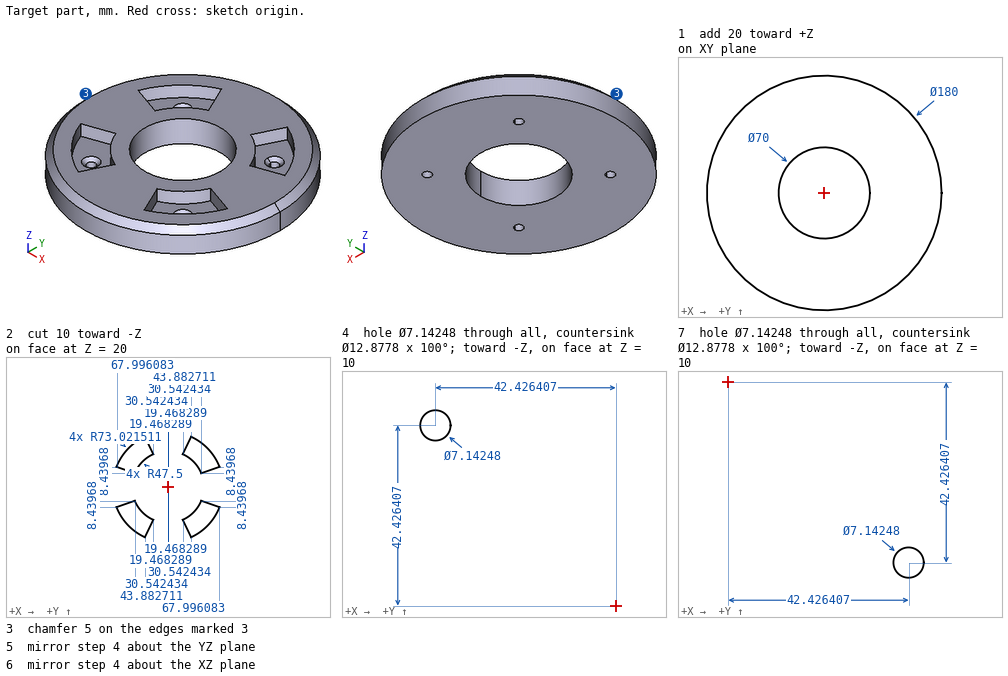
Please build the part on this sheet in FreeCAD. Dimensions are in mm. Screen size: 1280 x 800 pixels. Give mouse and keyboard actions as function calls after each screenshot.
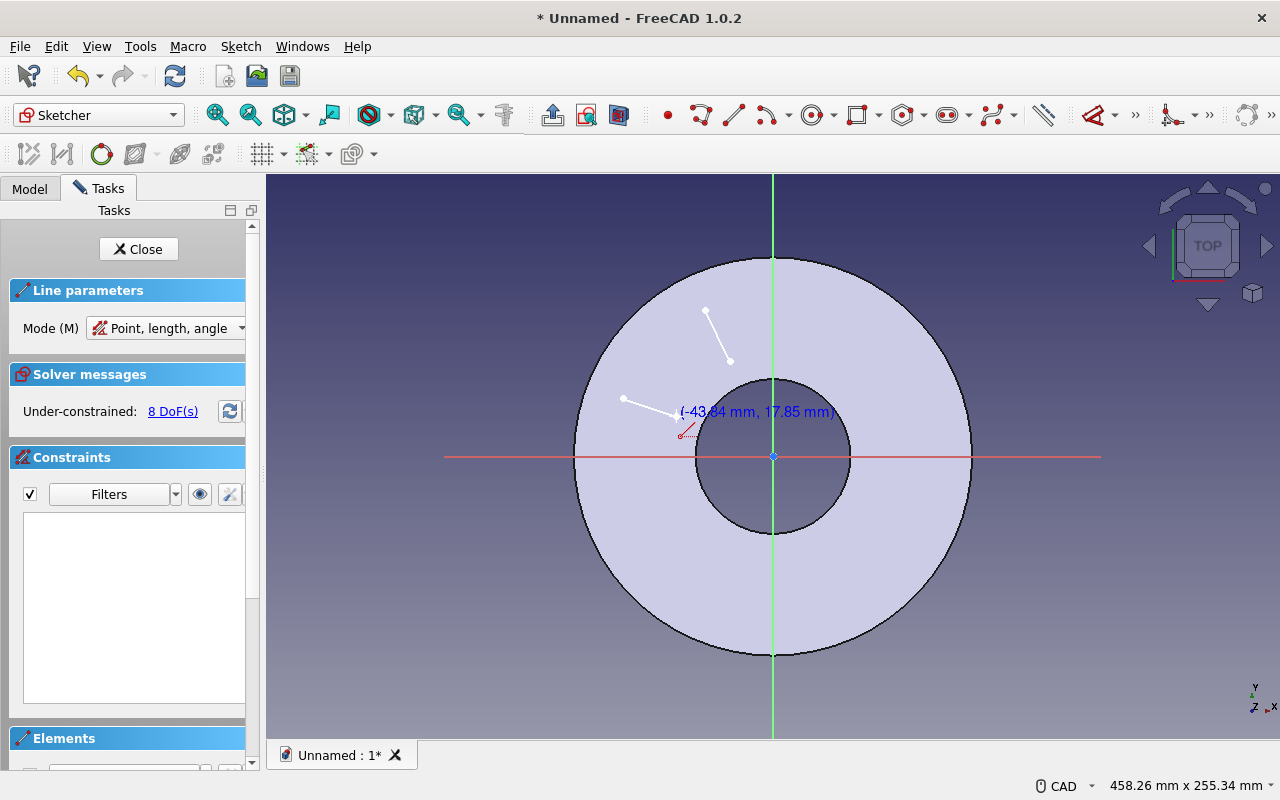
key(g)
key(3)
key(a)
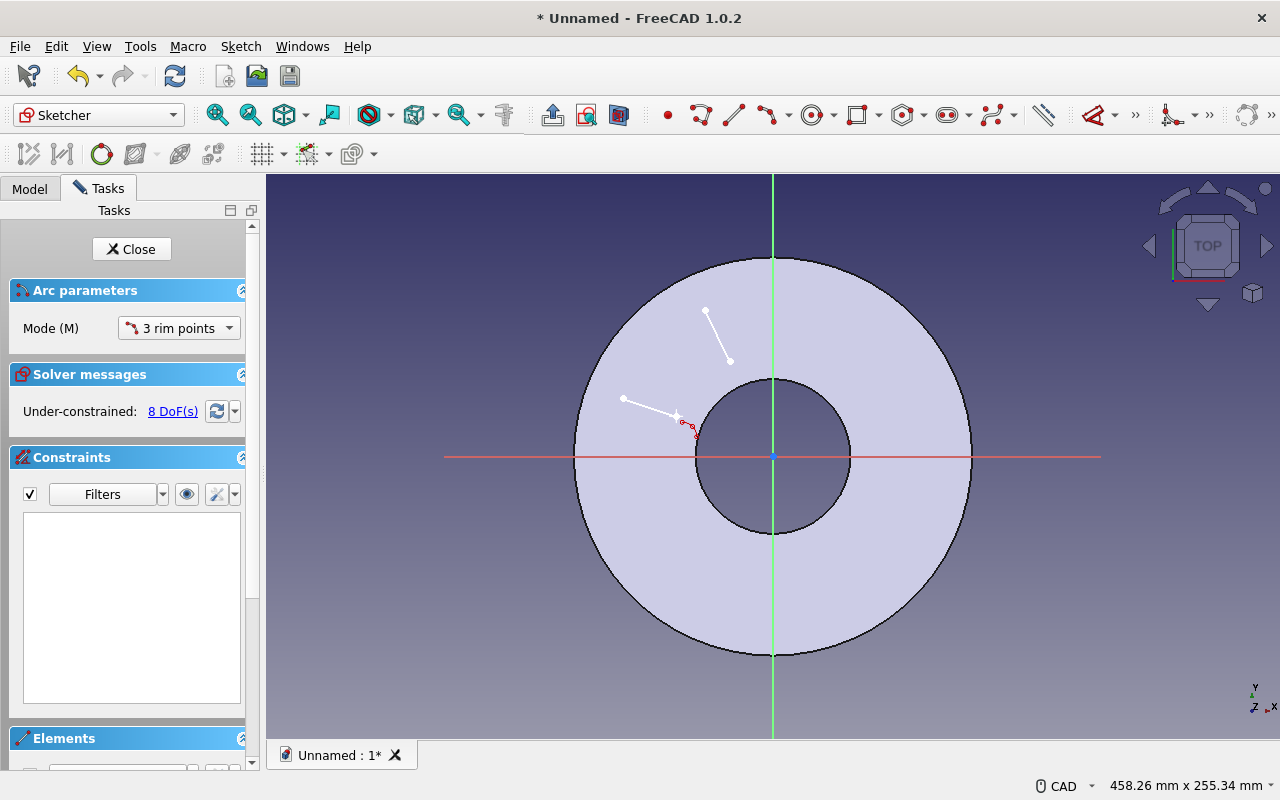
click(705, 311)
click(623, 399)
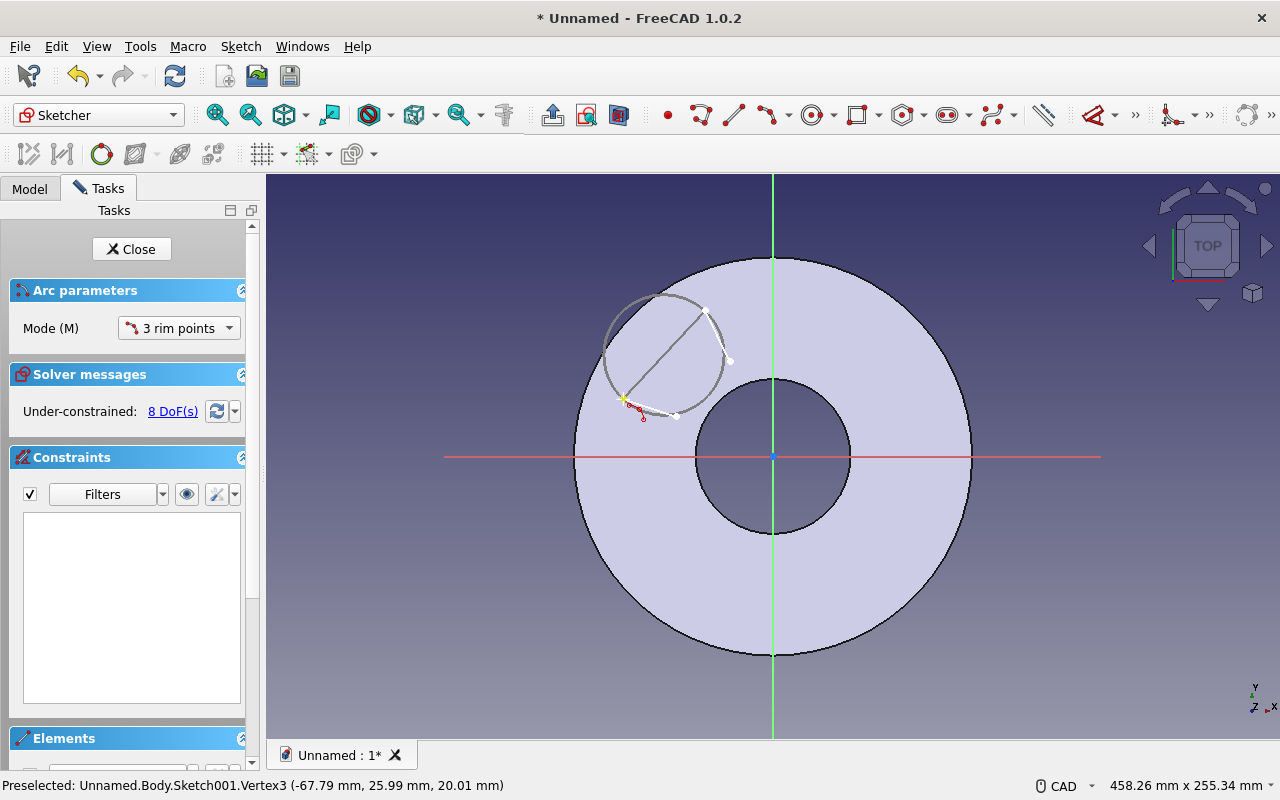
scroll(655, 346, up, 2)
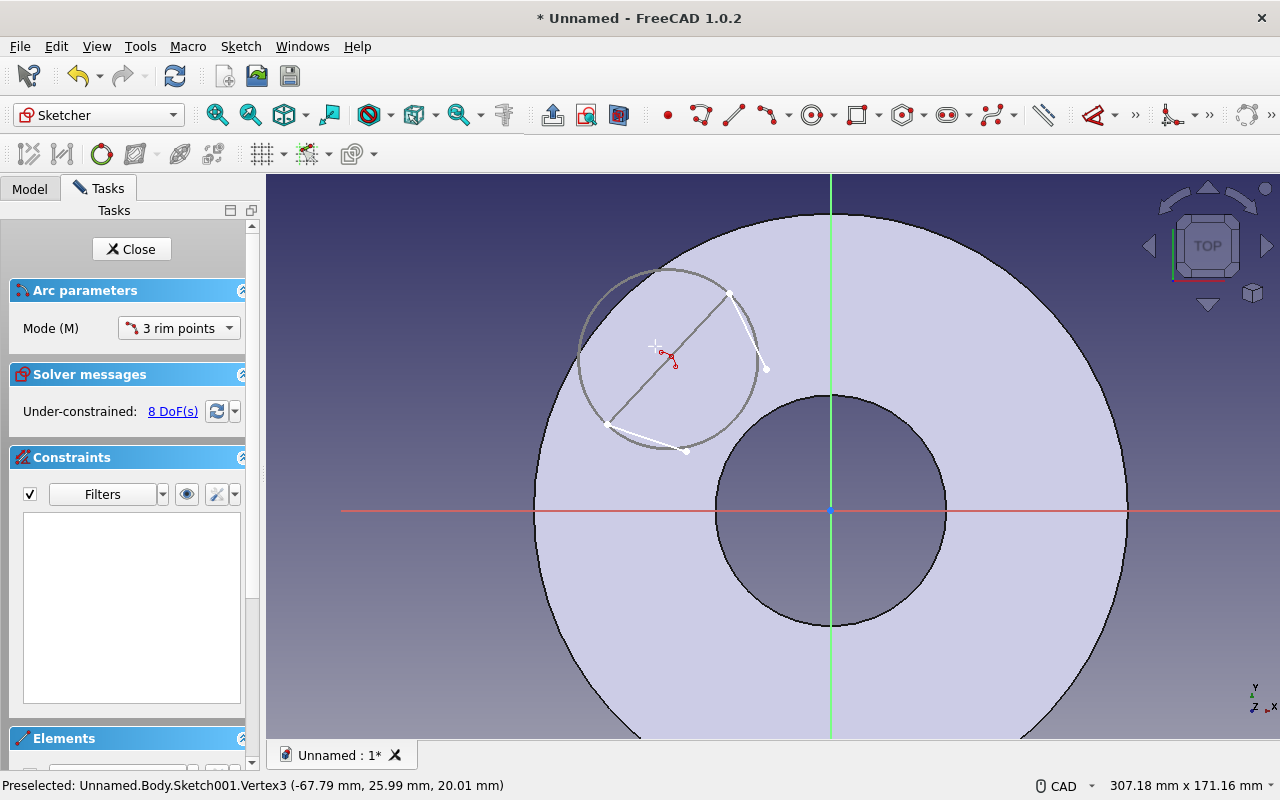
click(656, 345)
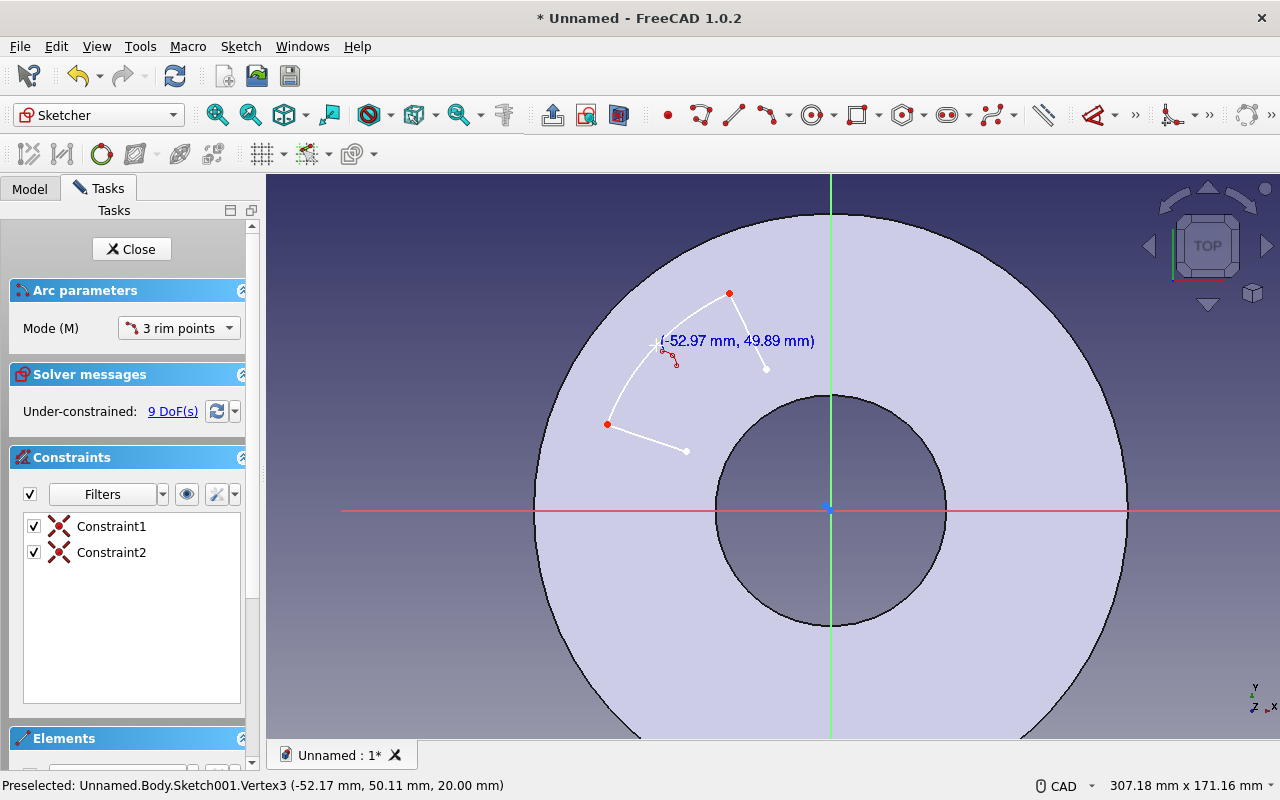
click(686, 452)
click(767, 370)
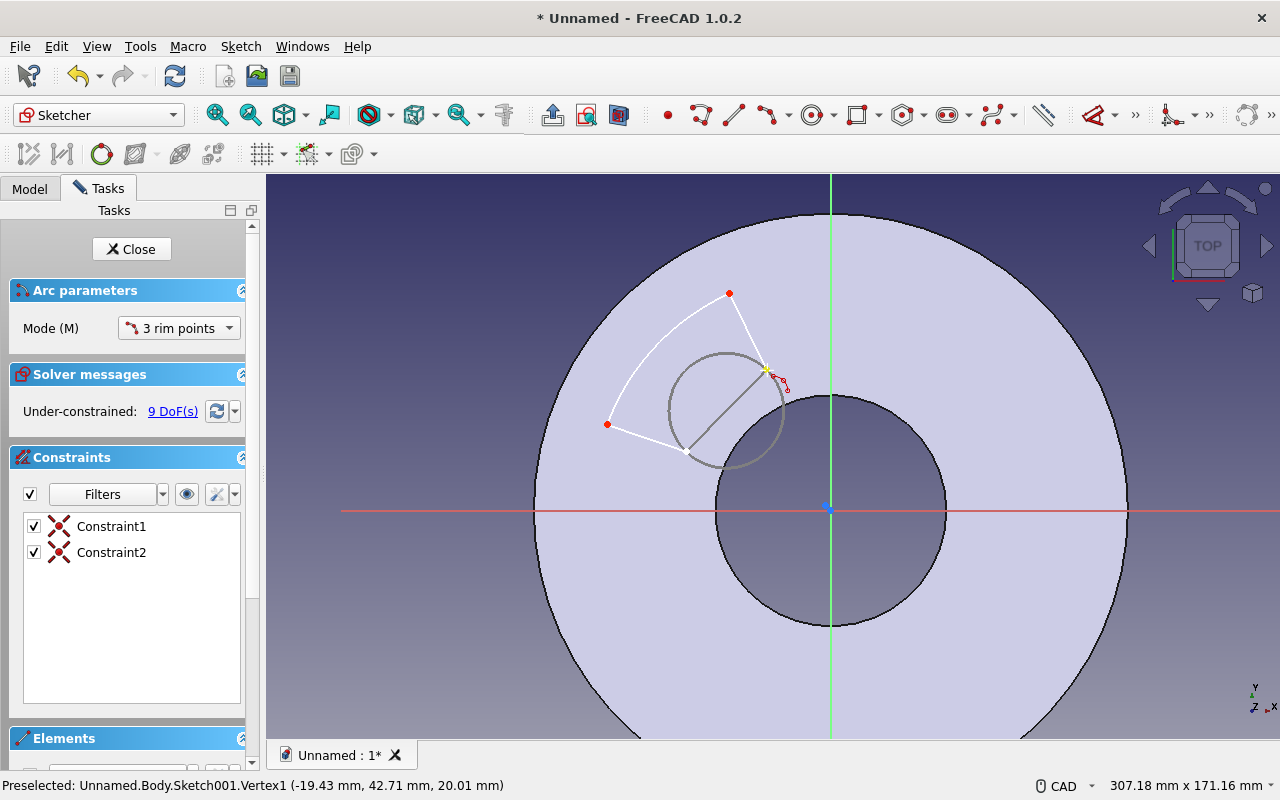
scroll(718, 401, up, 2)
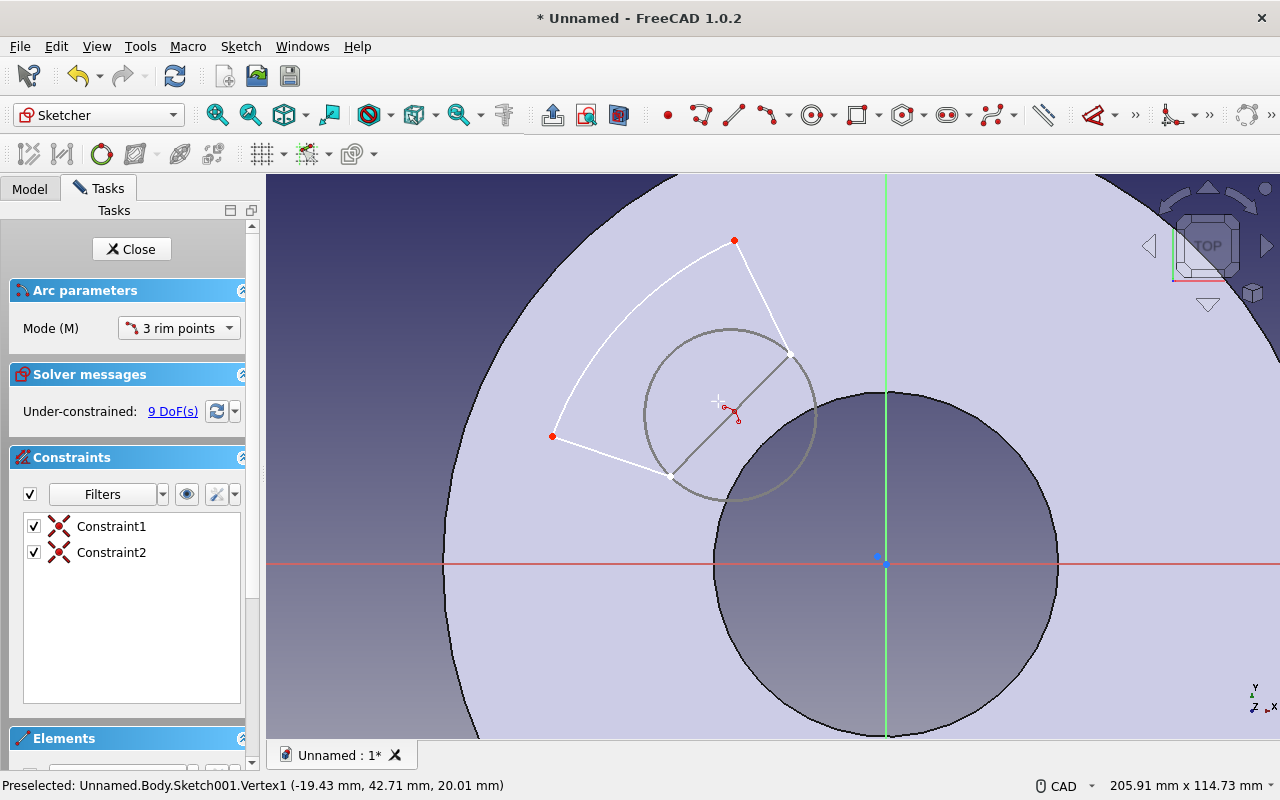
click(718, 402)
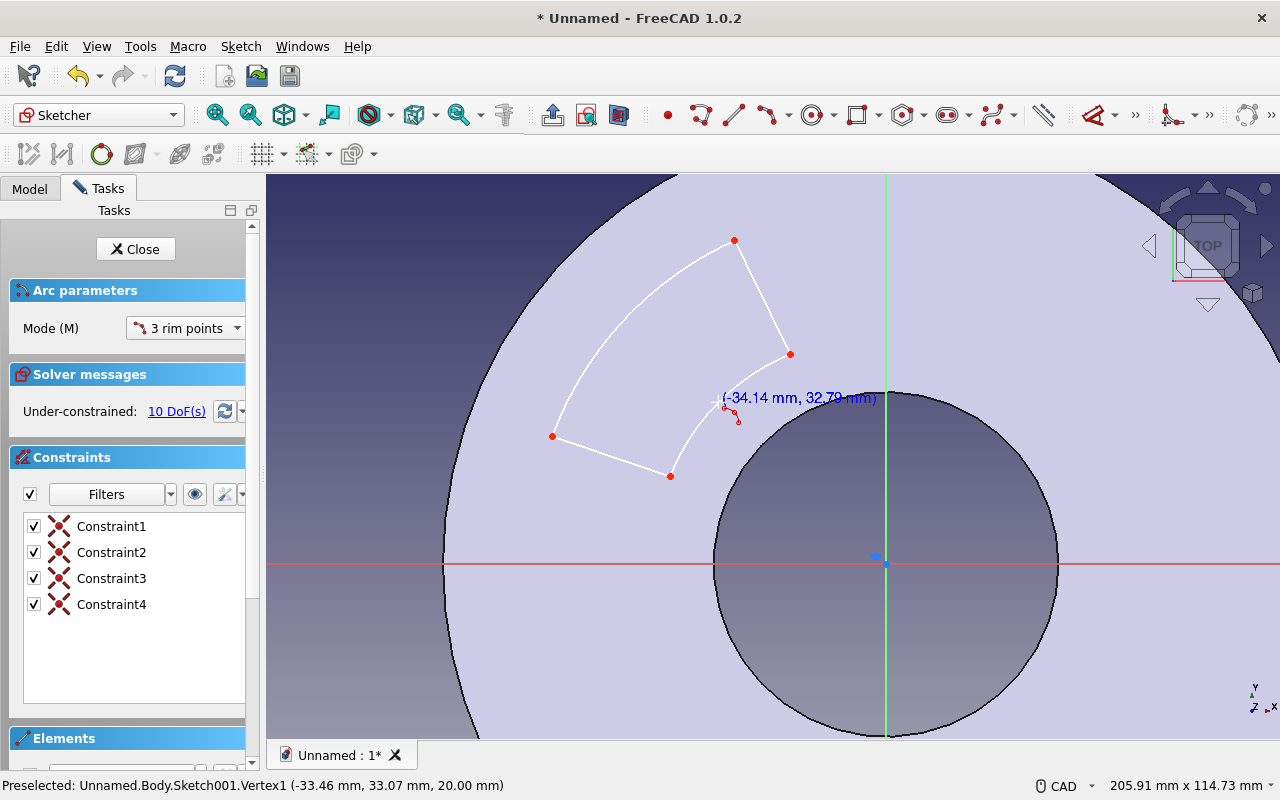
click(734, 116)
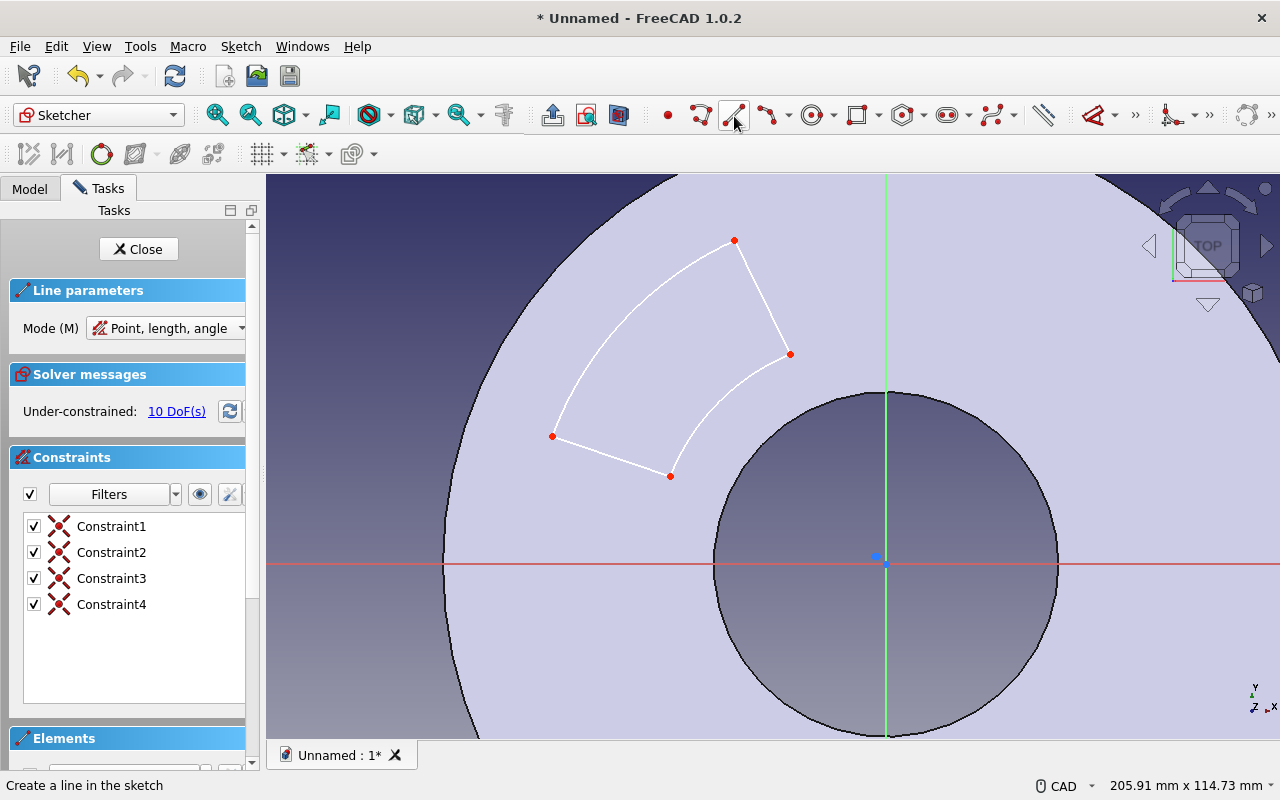
click(1102, 475)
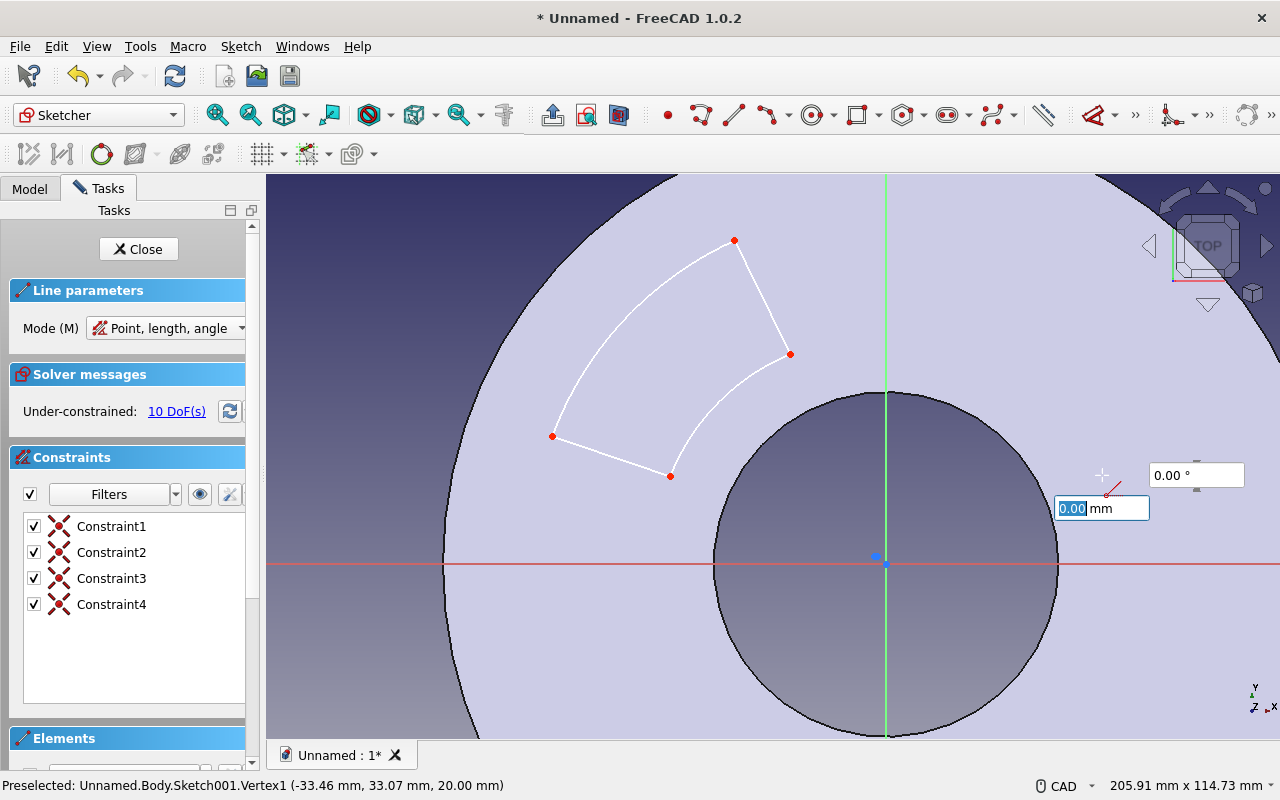
scroll(484, 325, down, 3)